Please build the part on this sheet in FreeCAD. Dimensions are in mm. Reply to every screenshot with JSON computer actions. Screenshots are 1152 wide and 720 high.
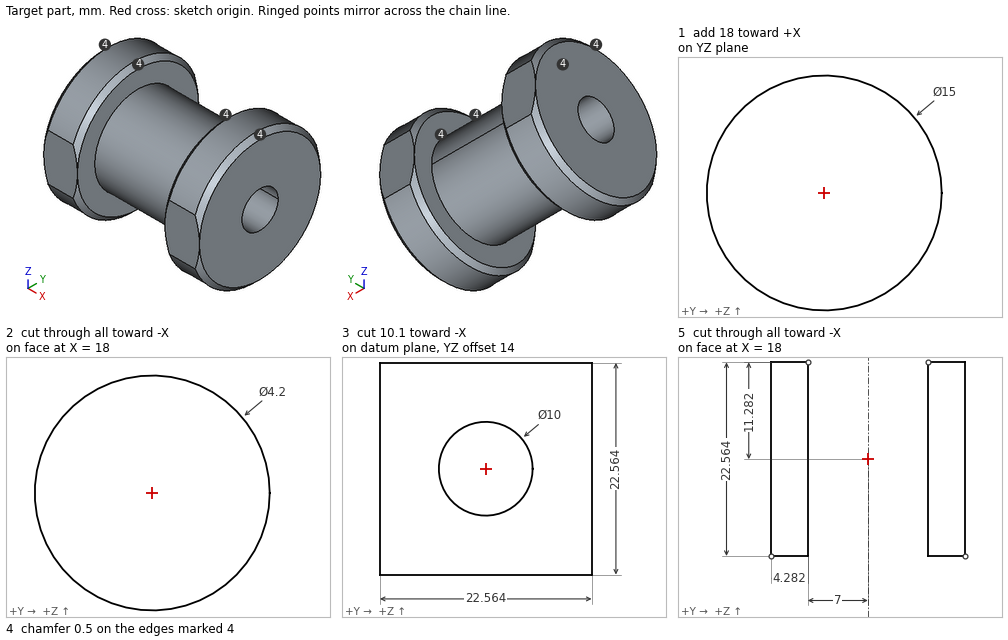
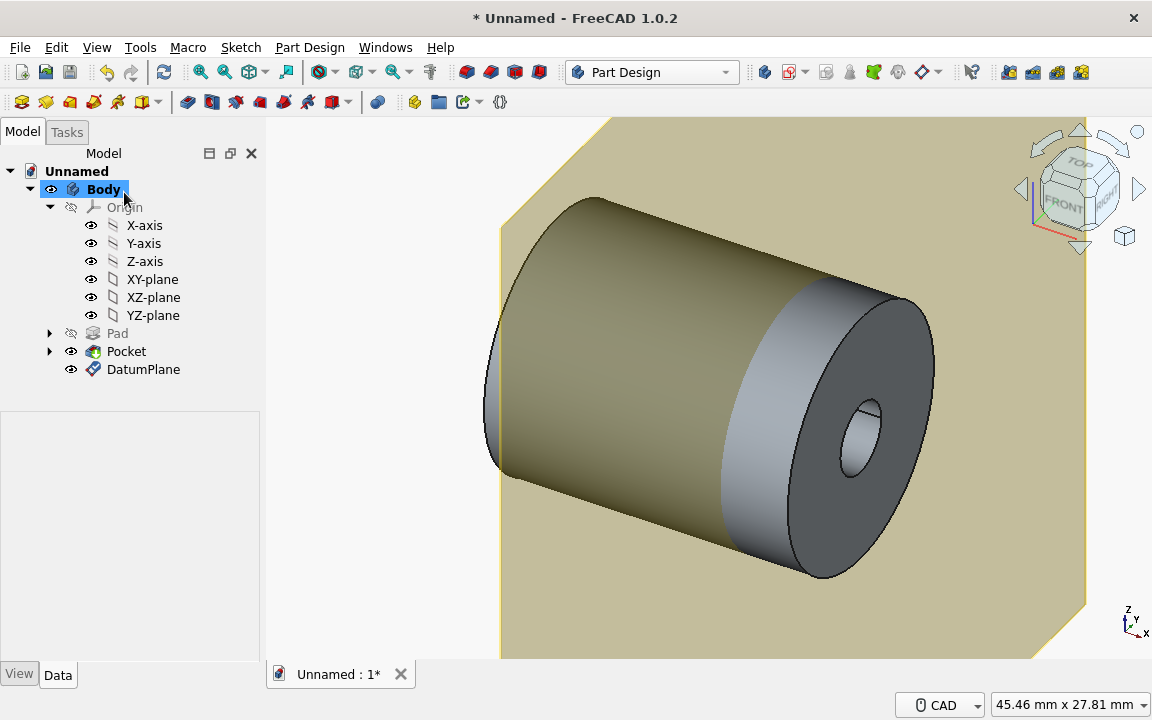
{"action": "left_click", "coordinate": [116, 369]}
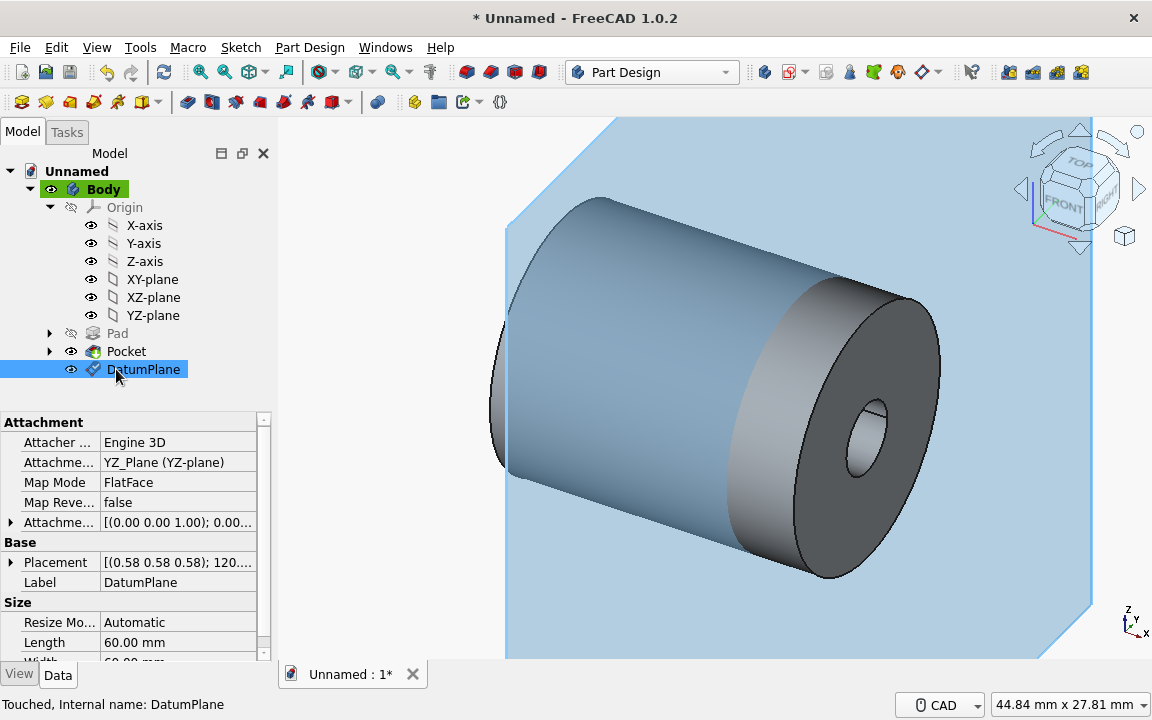
{"action": "left_click", "coordinate": [790, 72]}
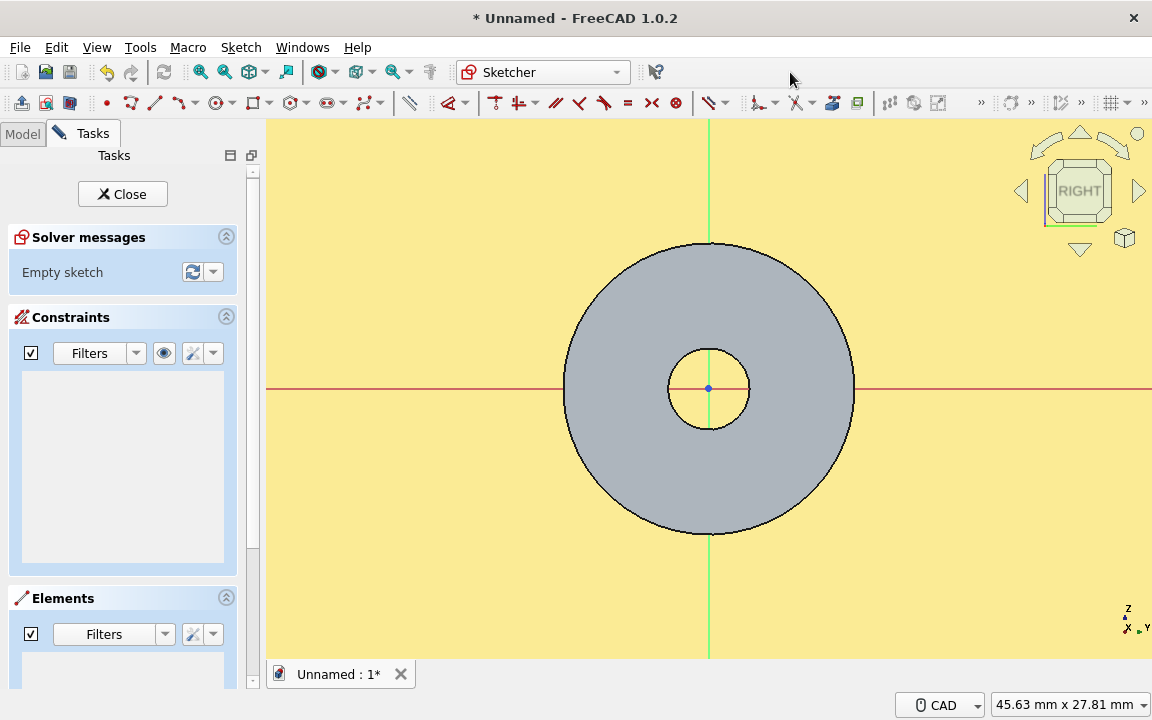
{"action": "key", "text": "q s"}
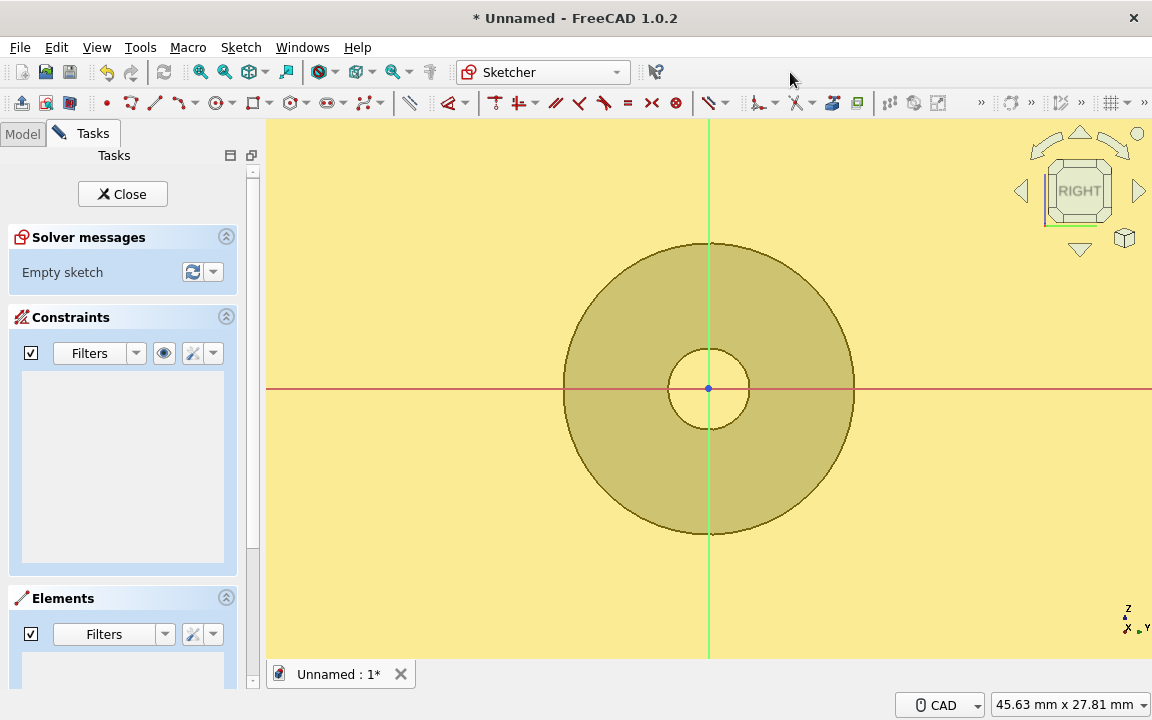
{"action": "scroll", "coordinate": [332, 389], "scroll_direction": "down", "scroll_amount": 1}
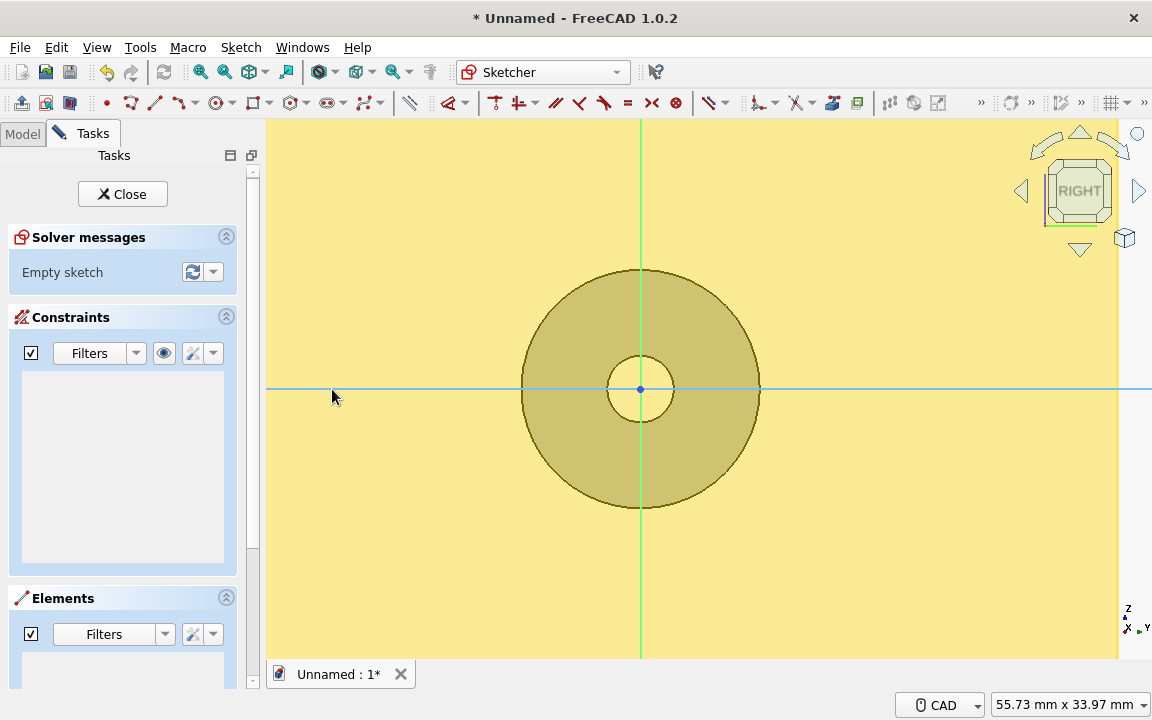
{"action": "key", "text": "g v"}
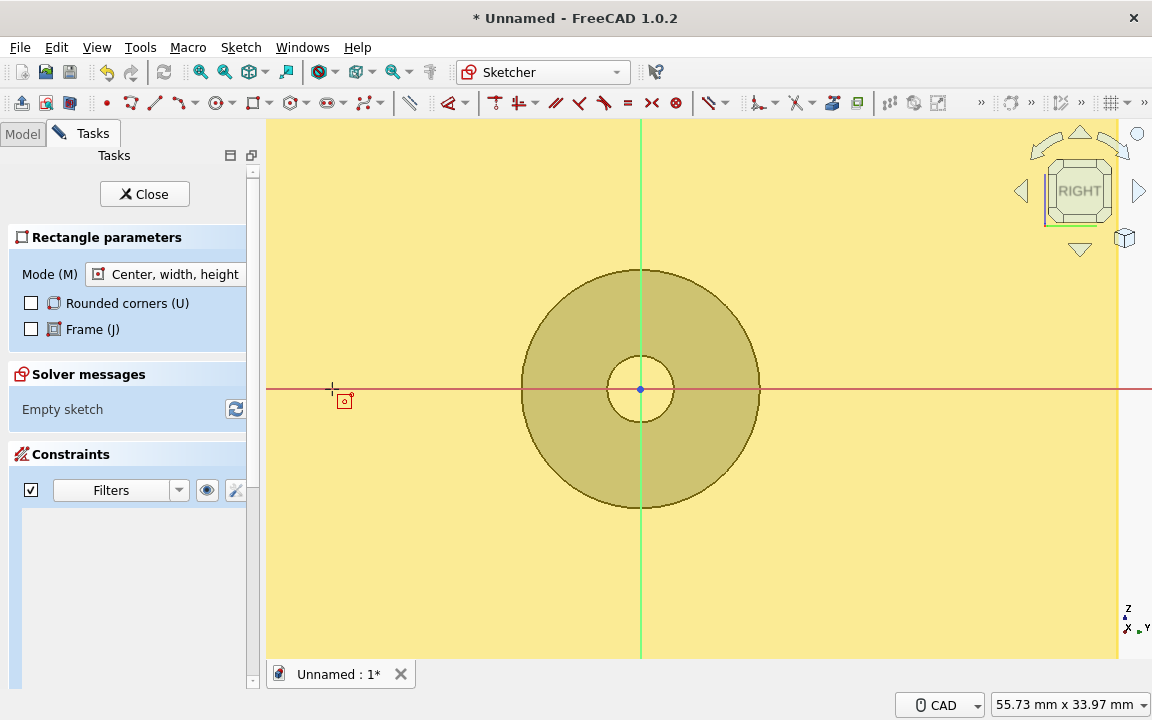
{"action": "left_click", "coordinate": [641, 389]}
{"action": "left_click", "coordinate": [820, 210]}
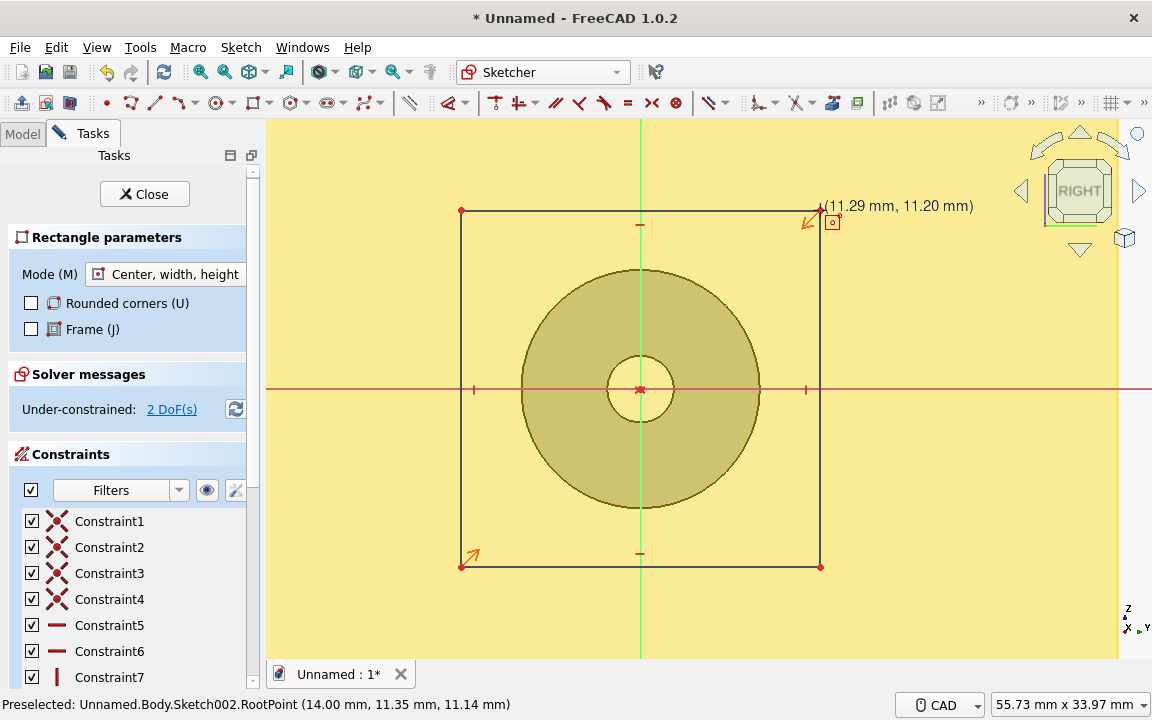
{"action": "left_click", "coordinate": [216, 104]}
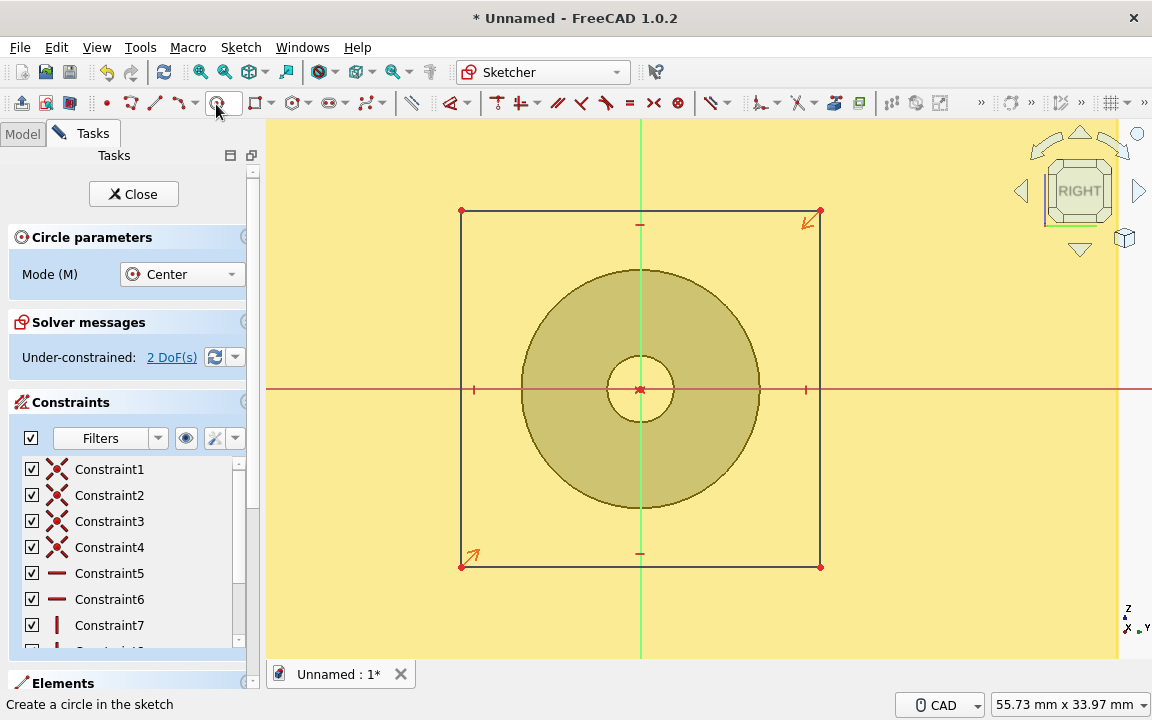
{"action": "left_click", "coordinate": [641, 389]}
{"action": "left_click", "coordinate": [697, 333]}
{"action": "key", "text": "Escape"}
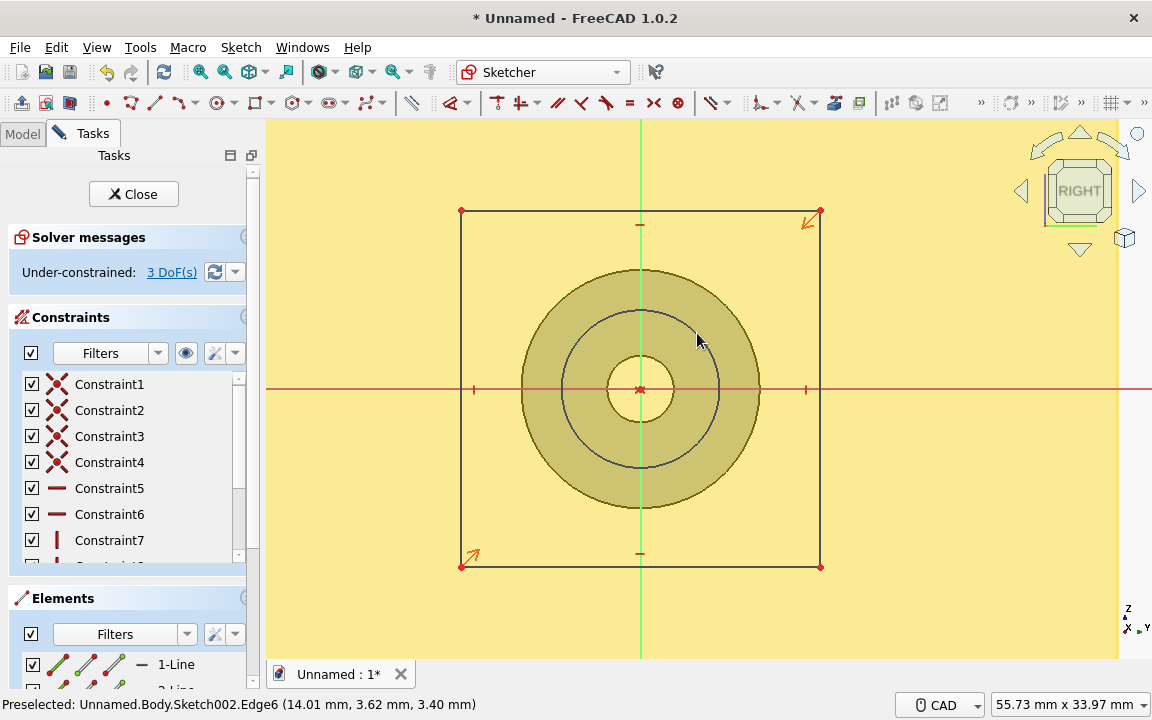
{"action": "left_click", "coordinate": [450, 104]}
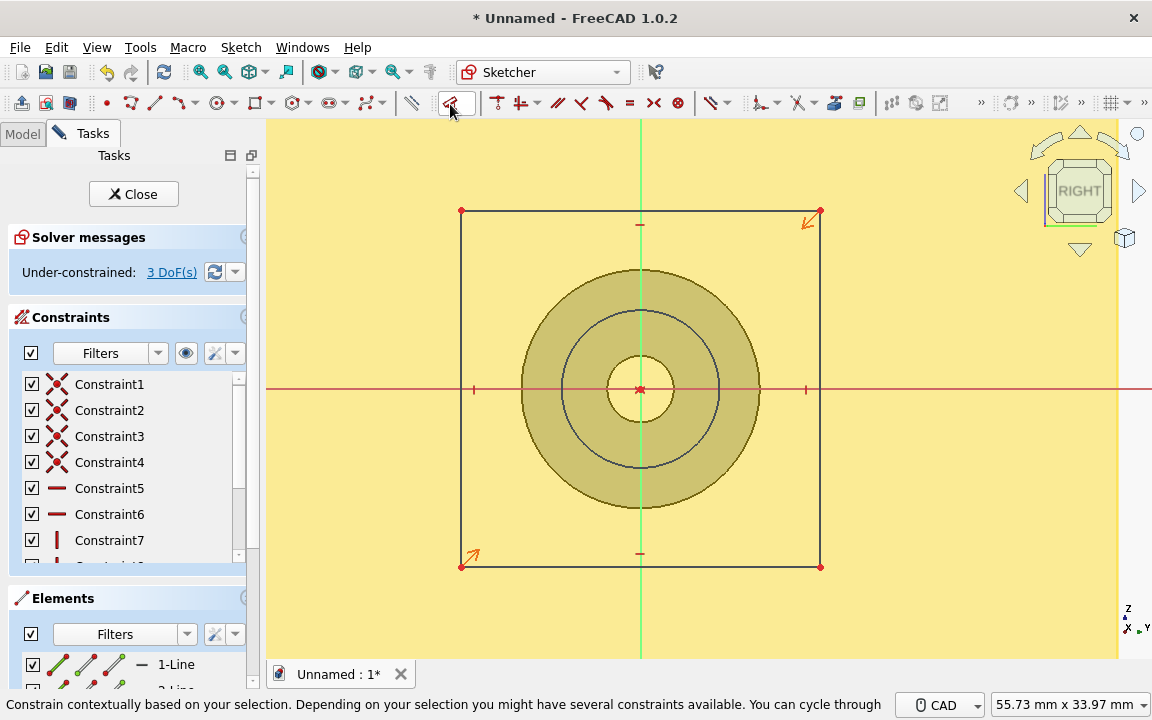
{"action": "left_click", "coordinate": [696, 333]}
{"action": "left_click", "coordinate": [718, 310]}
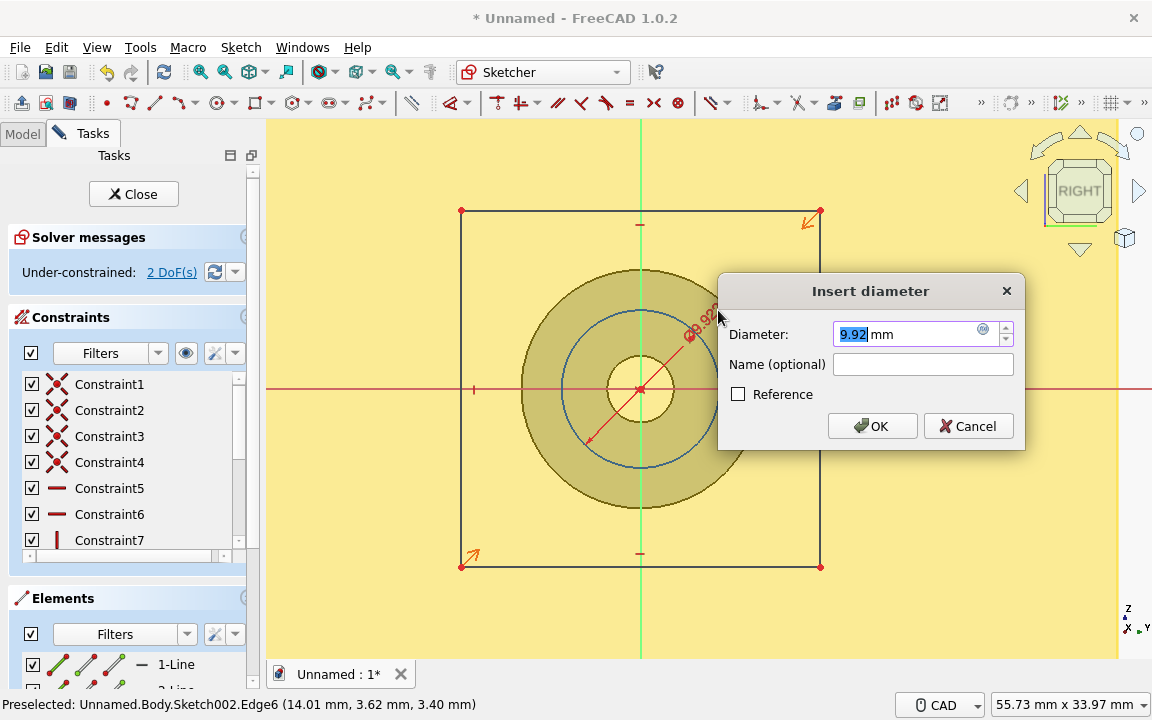
{"action": "type", "text": "10"}
{"action": "key", "text": "Return"}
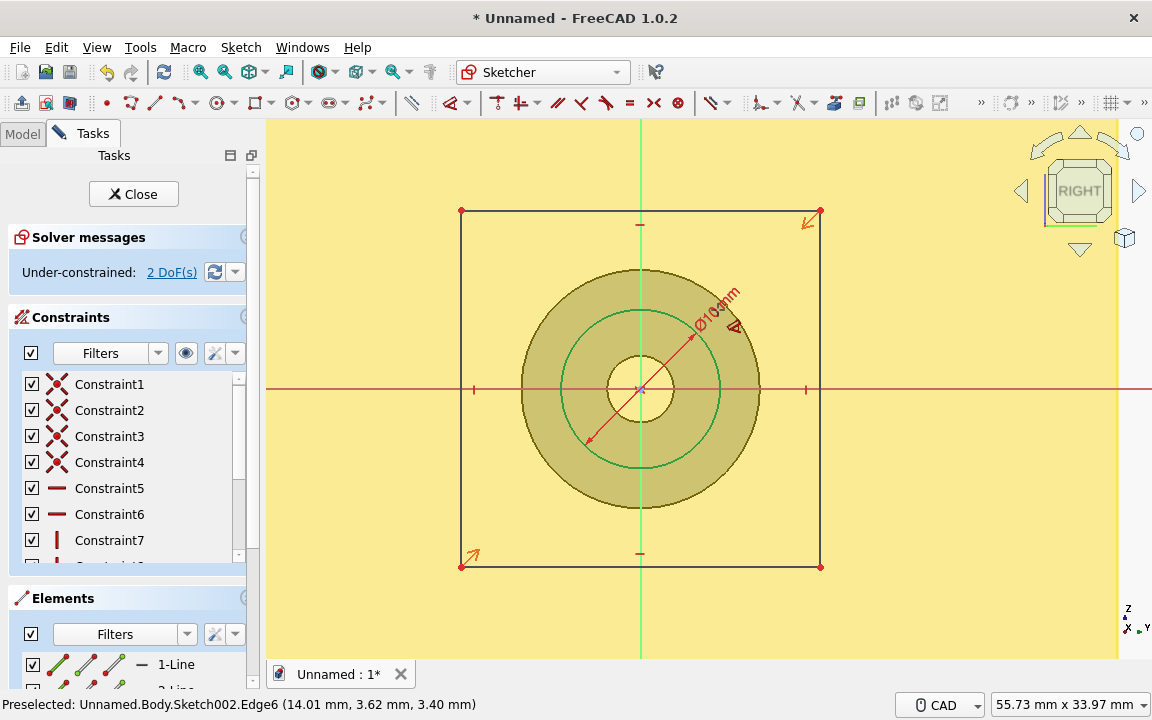
{"action": "left_click", "coordinate": [569, 567]}
{"action": "left_click", "coordinate": [558, 601]}